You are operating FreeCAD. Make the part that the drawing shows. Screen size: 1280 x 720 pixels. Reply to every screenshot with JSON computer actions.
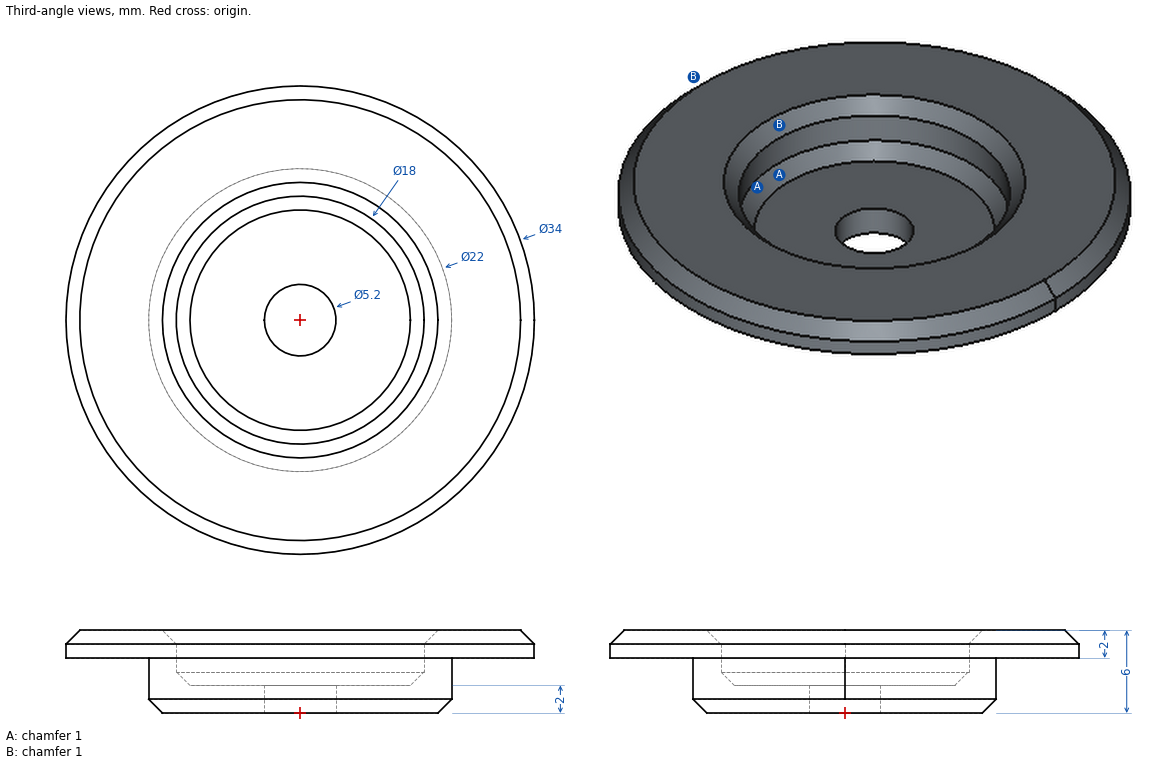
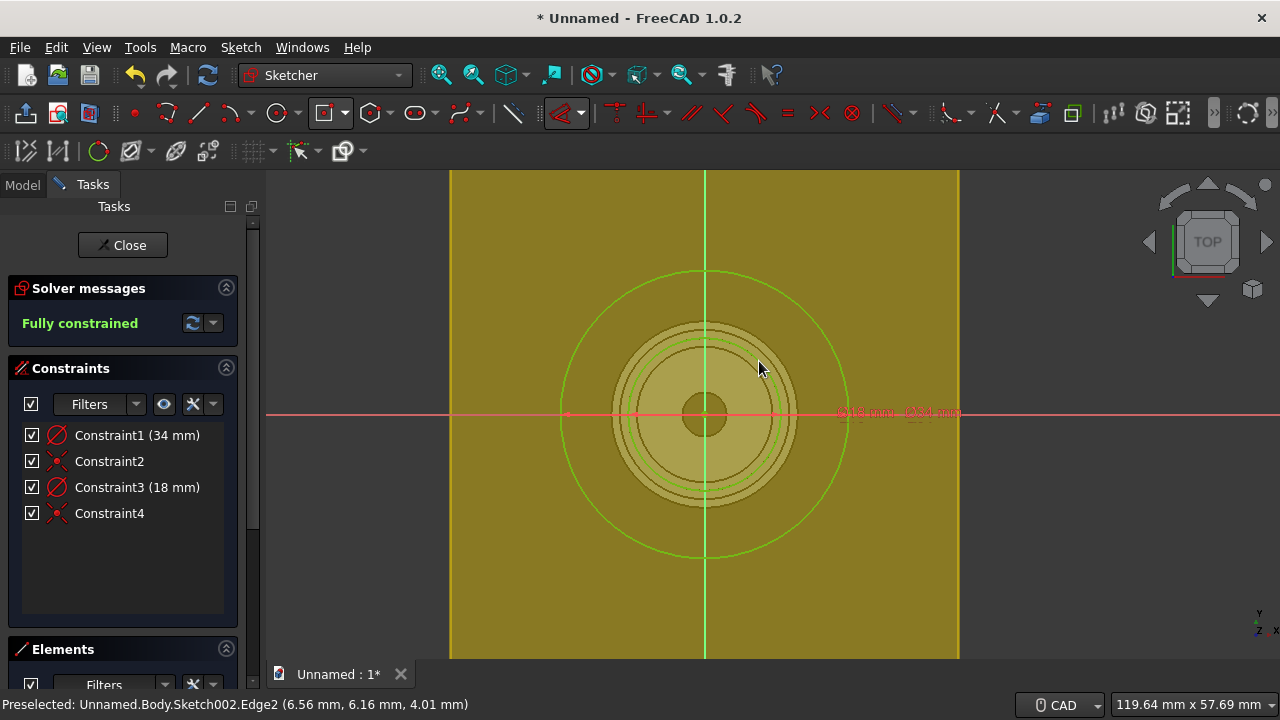
{"action": "left_click", "coordinate": [123, 245]}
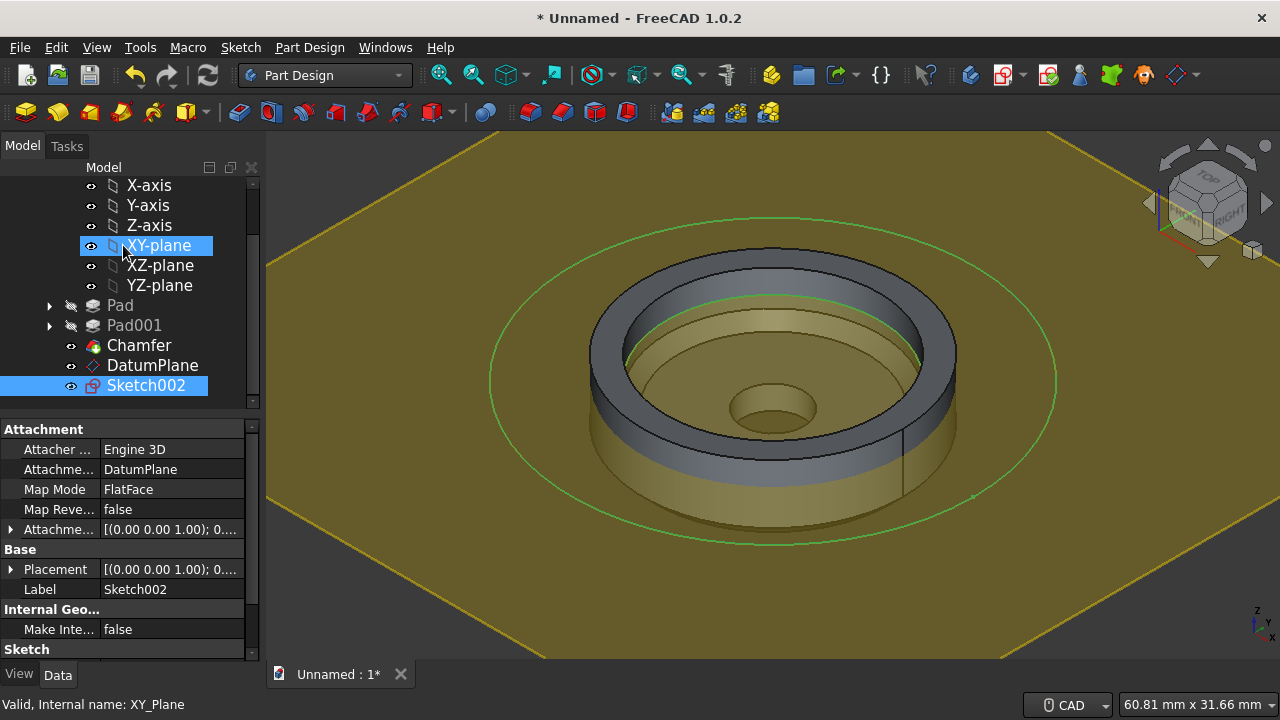
{"action": "left_click", "coordinate": [26, 112]}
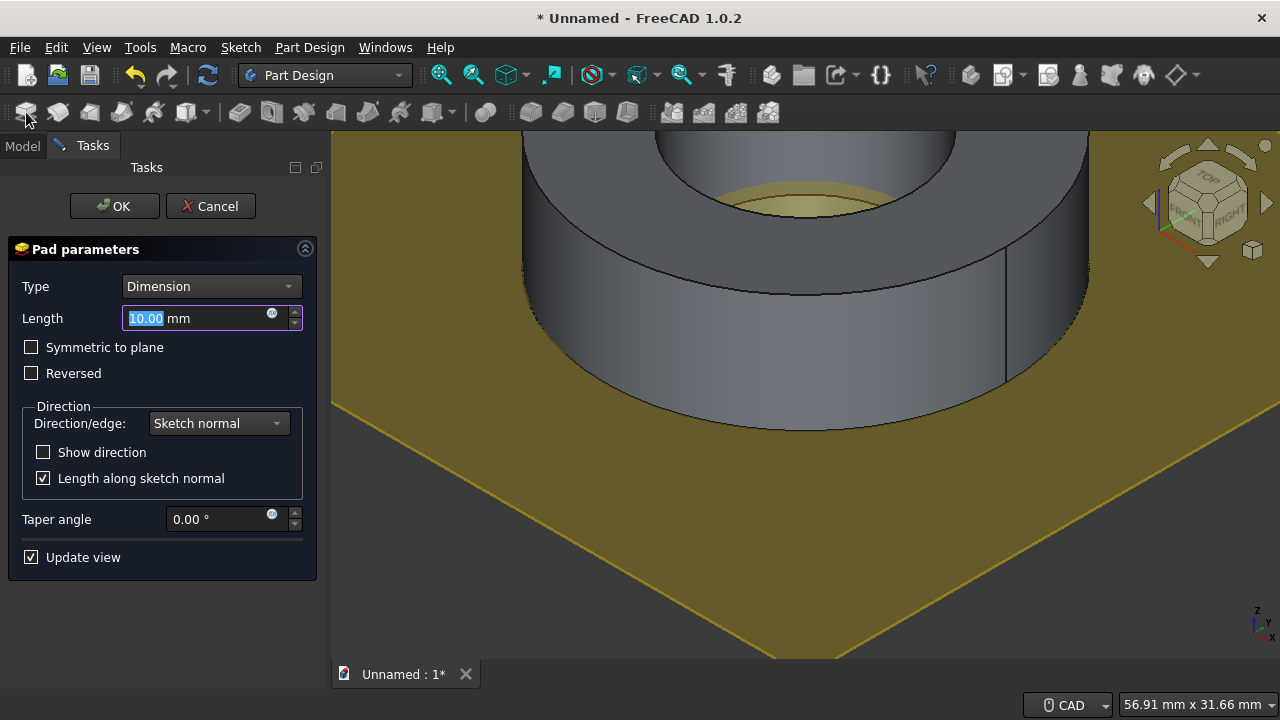
{"action": "type", "text": "2"}
{"action": "key", "text": "Tab"}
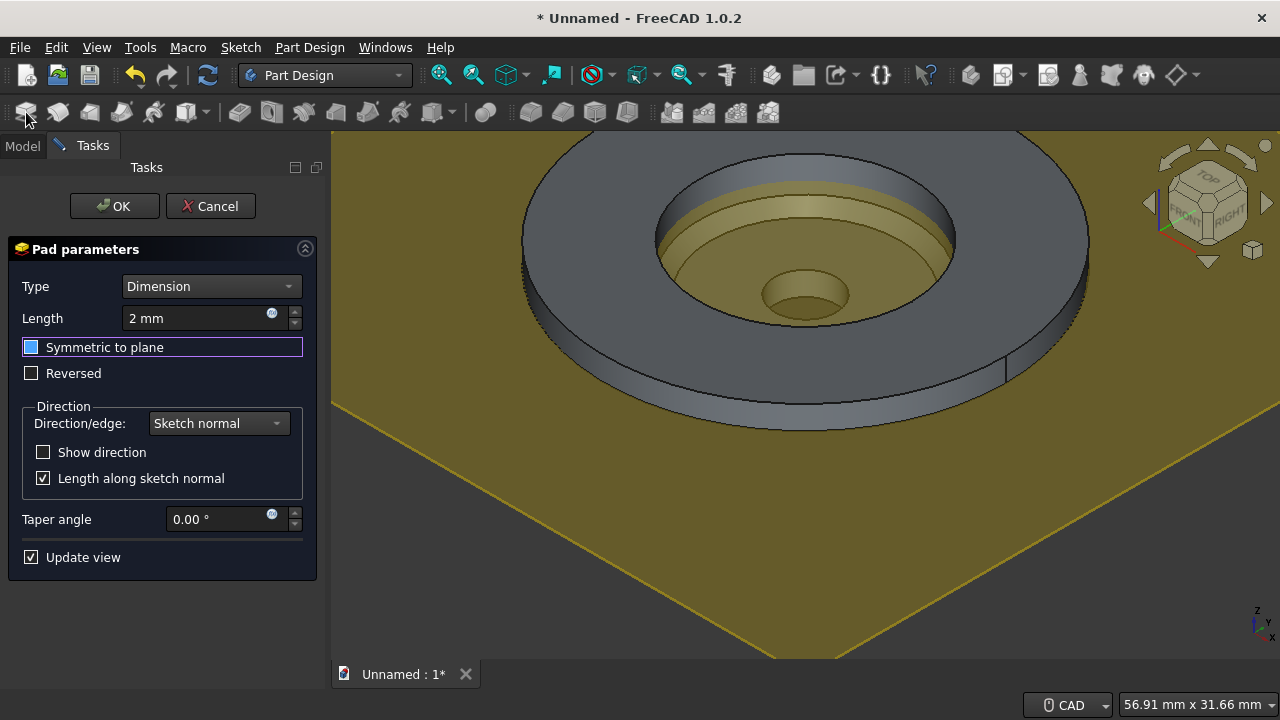
{"action": "left_click", "coordinate": [115, 206]}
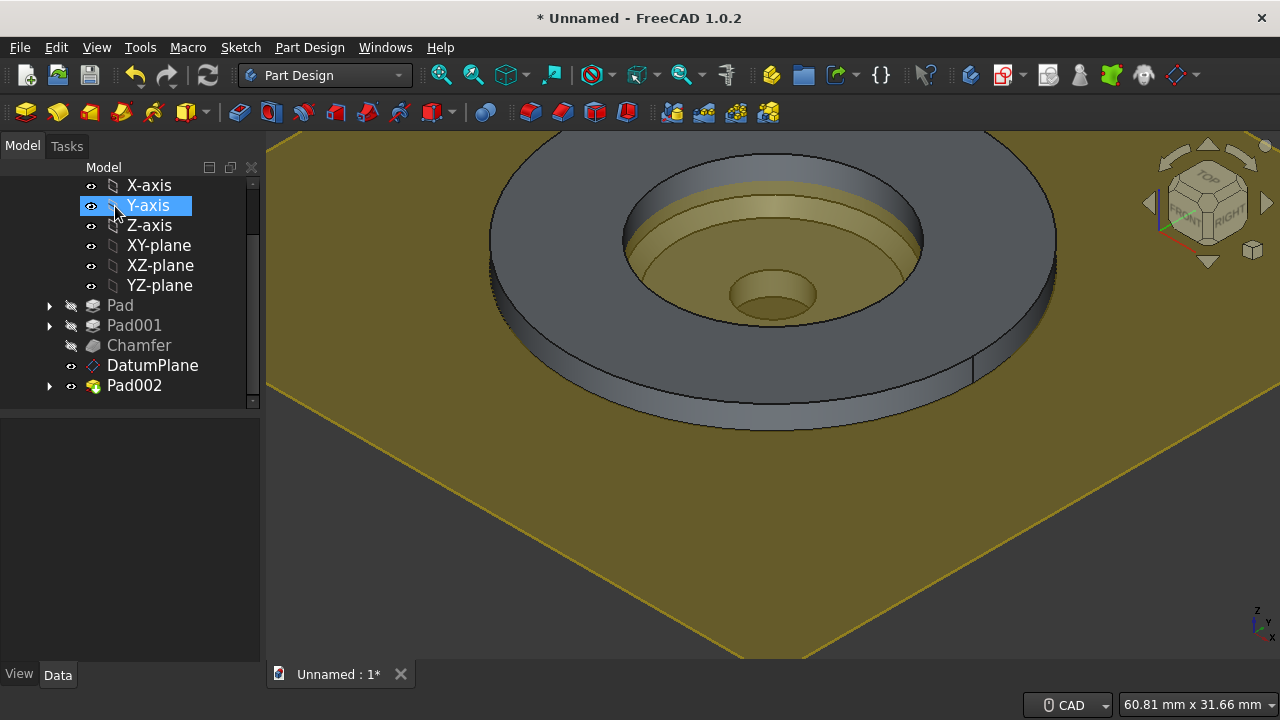
{"action": "left_click", "coordinate": [116, 366]}
{"action": "key", "text": "space"}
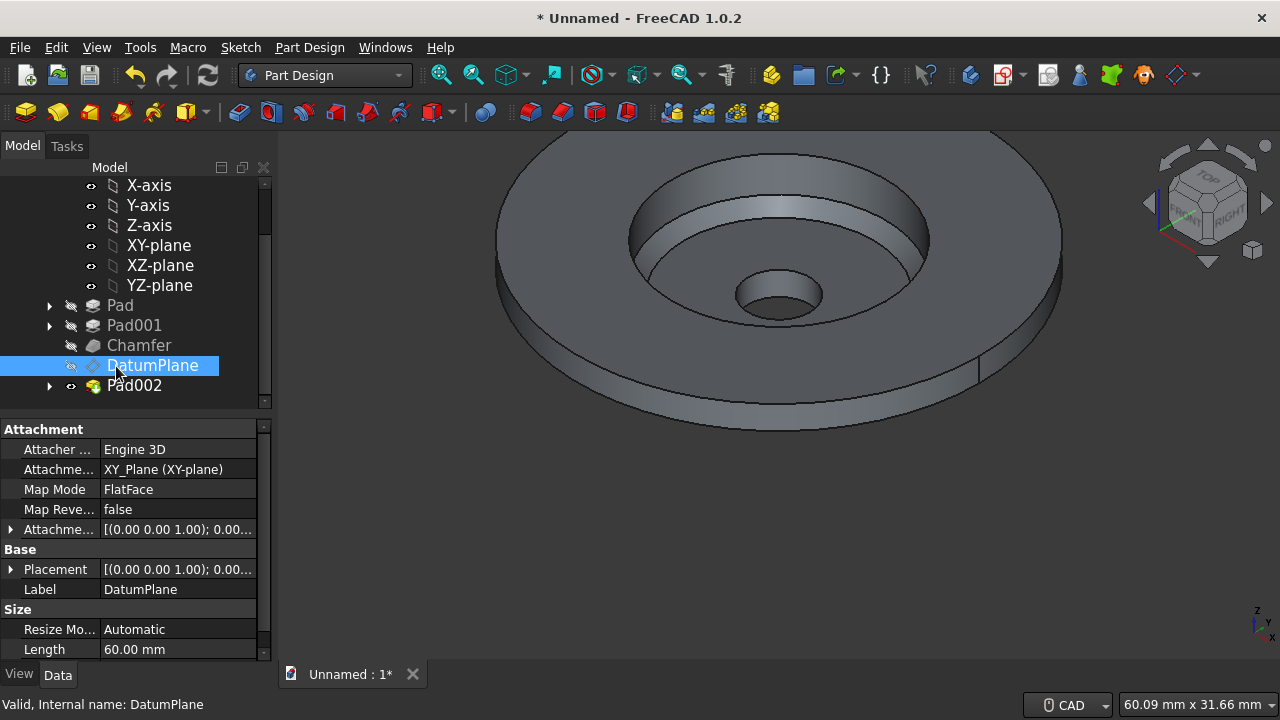
{"action": "left_click", "coordinate": [442, 76]}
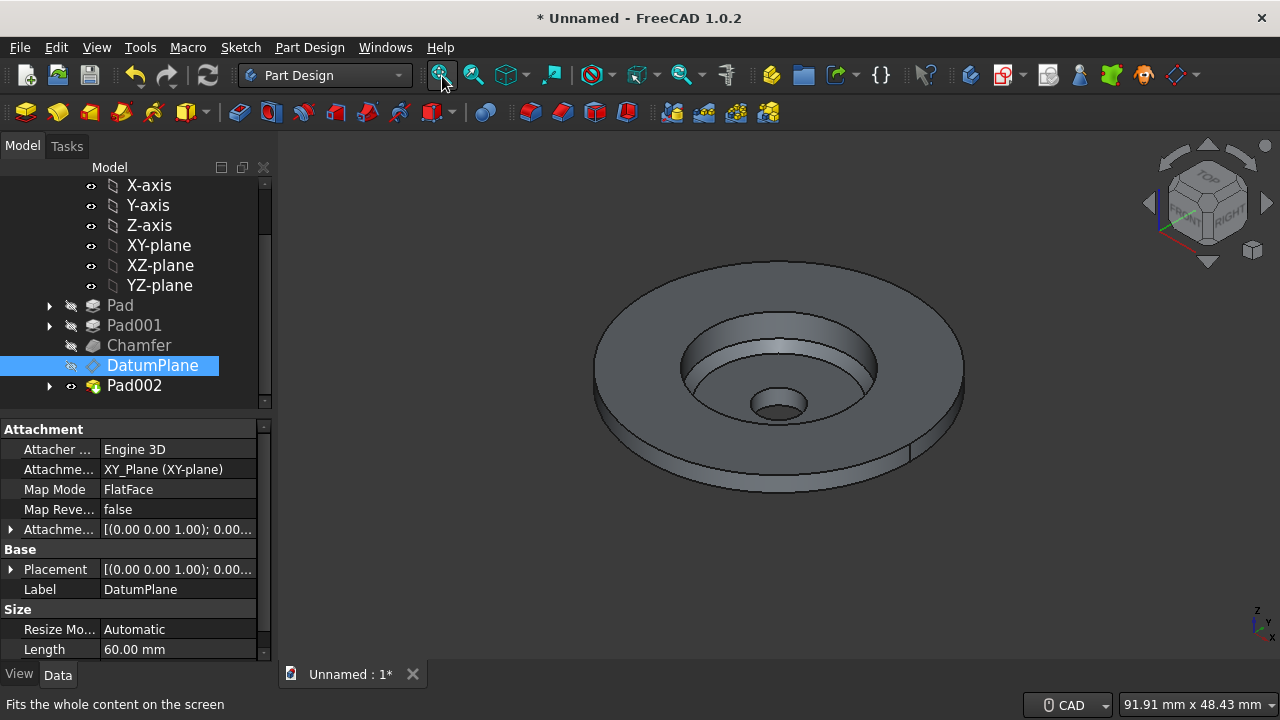
{"action": "left_click", "coordinate": [614, 416]}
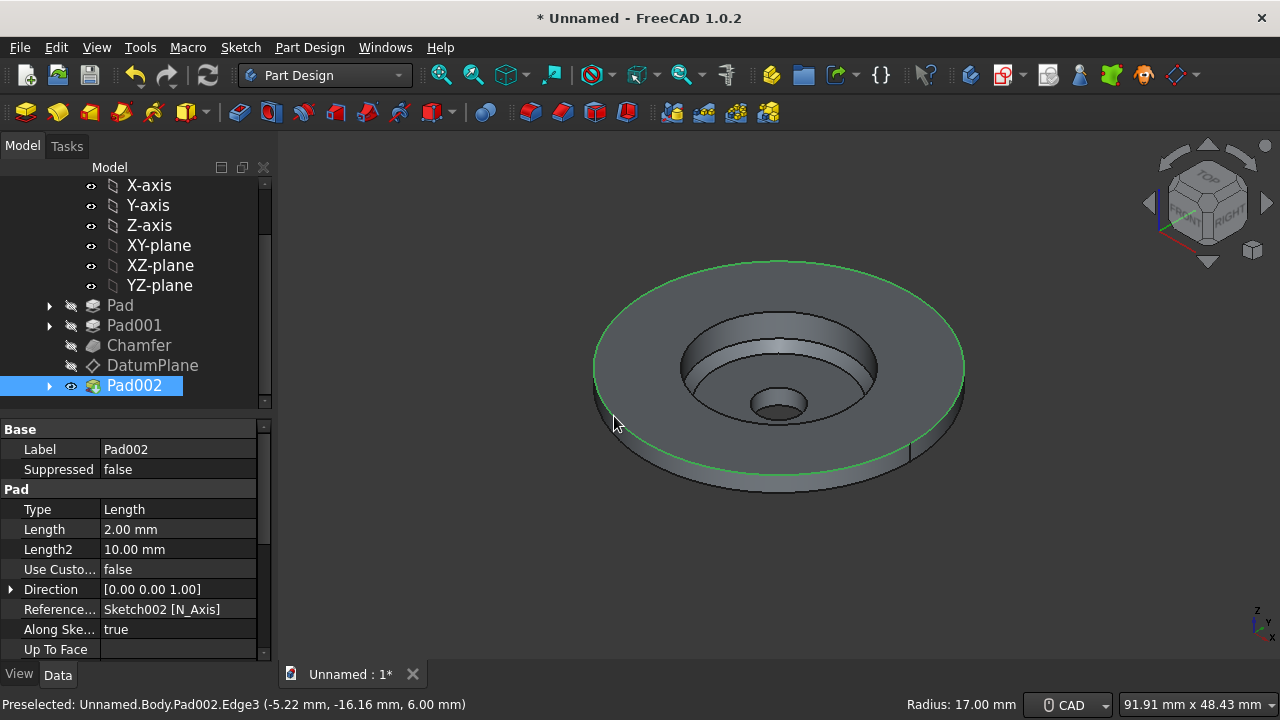
{"action": "left_click", "coordinate": [710, 327], "text": "ctrl"}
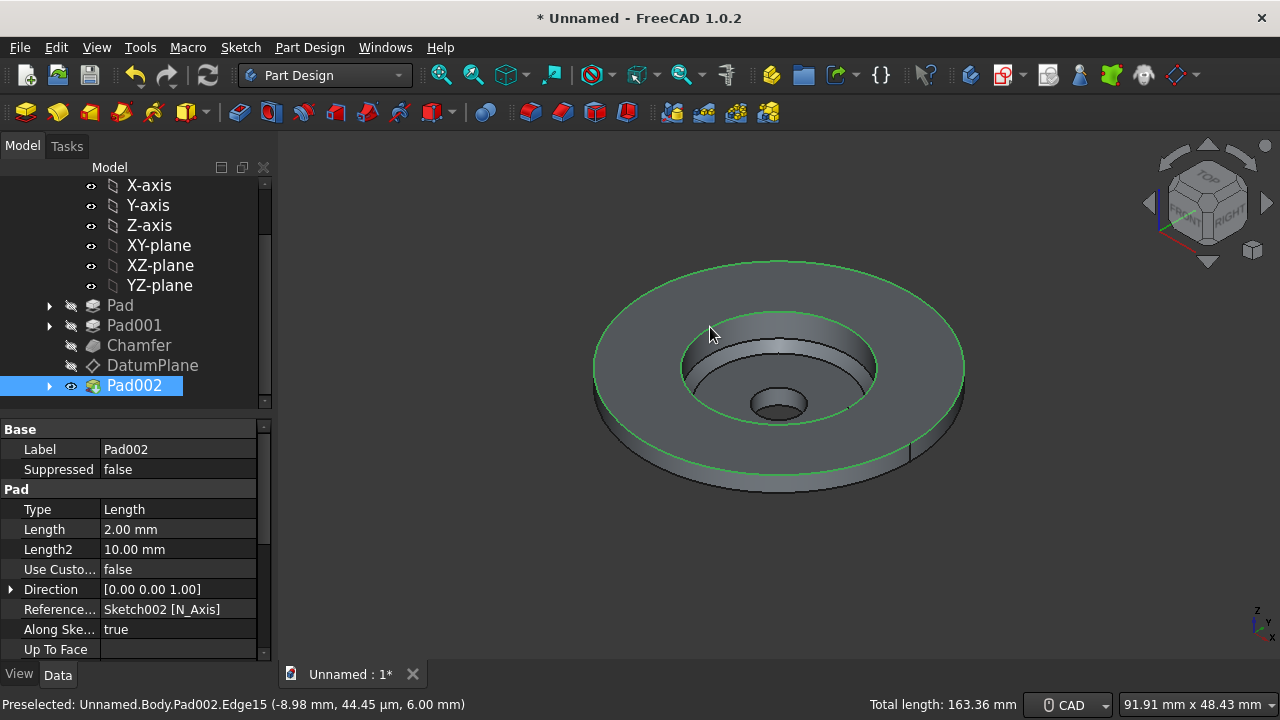
{"action": "left_click", "coordinate": [564, 112]}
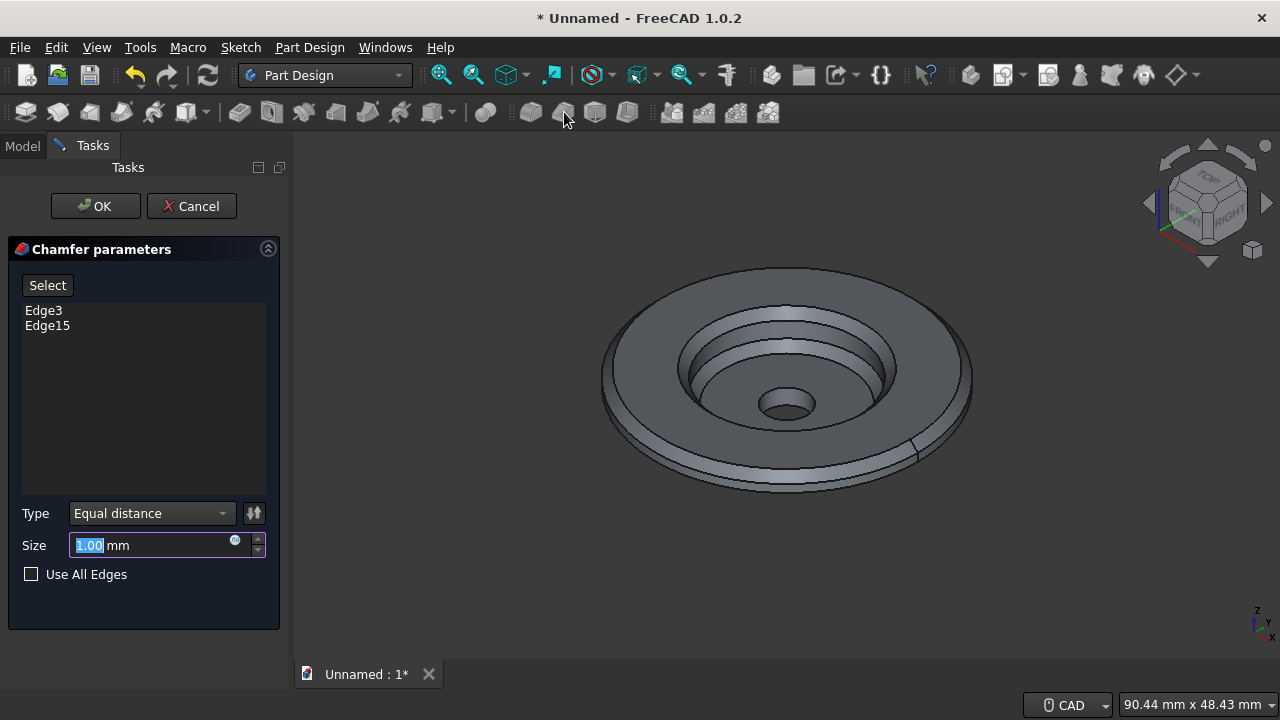
{"action": "type", "text": "1"}
{"action": "key", "text": "Tab"}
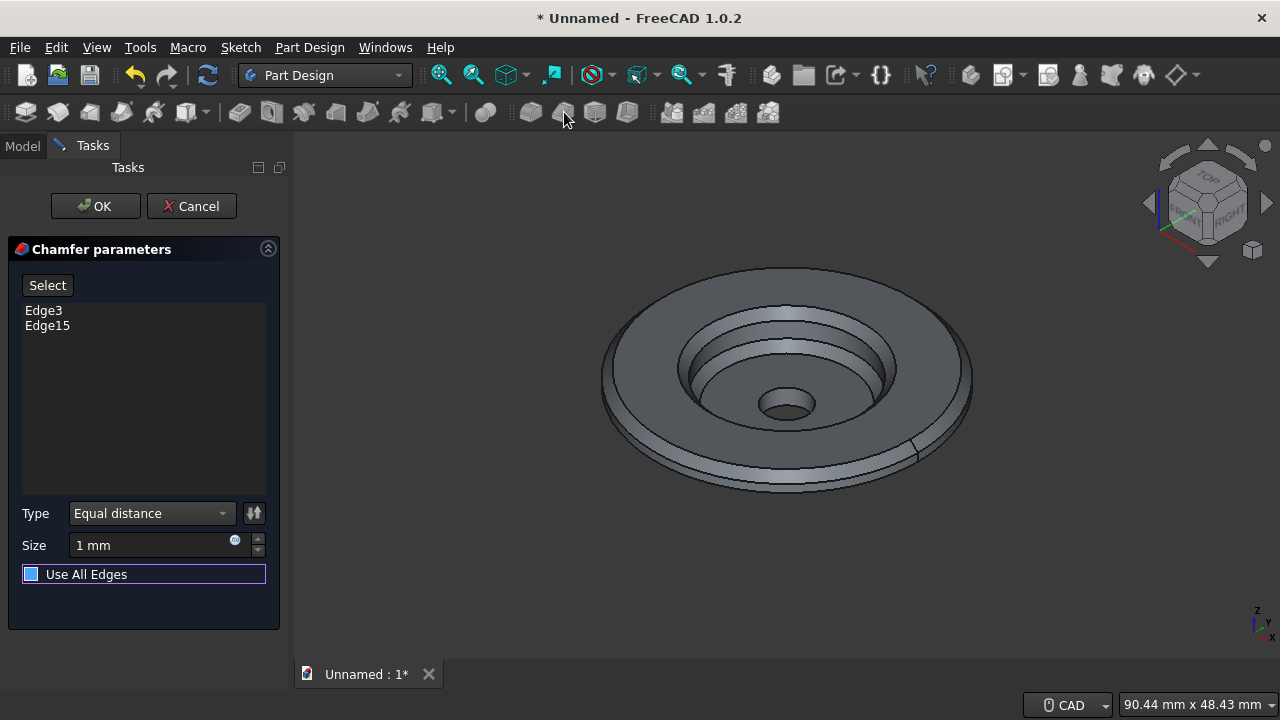
{"action": "left_click", "coordinate": [96, 206]}